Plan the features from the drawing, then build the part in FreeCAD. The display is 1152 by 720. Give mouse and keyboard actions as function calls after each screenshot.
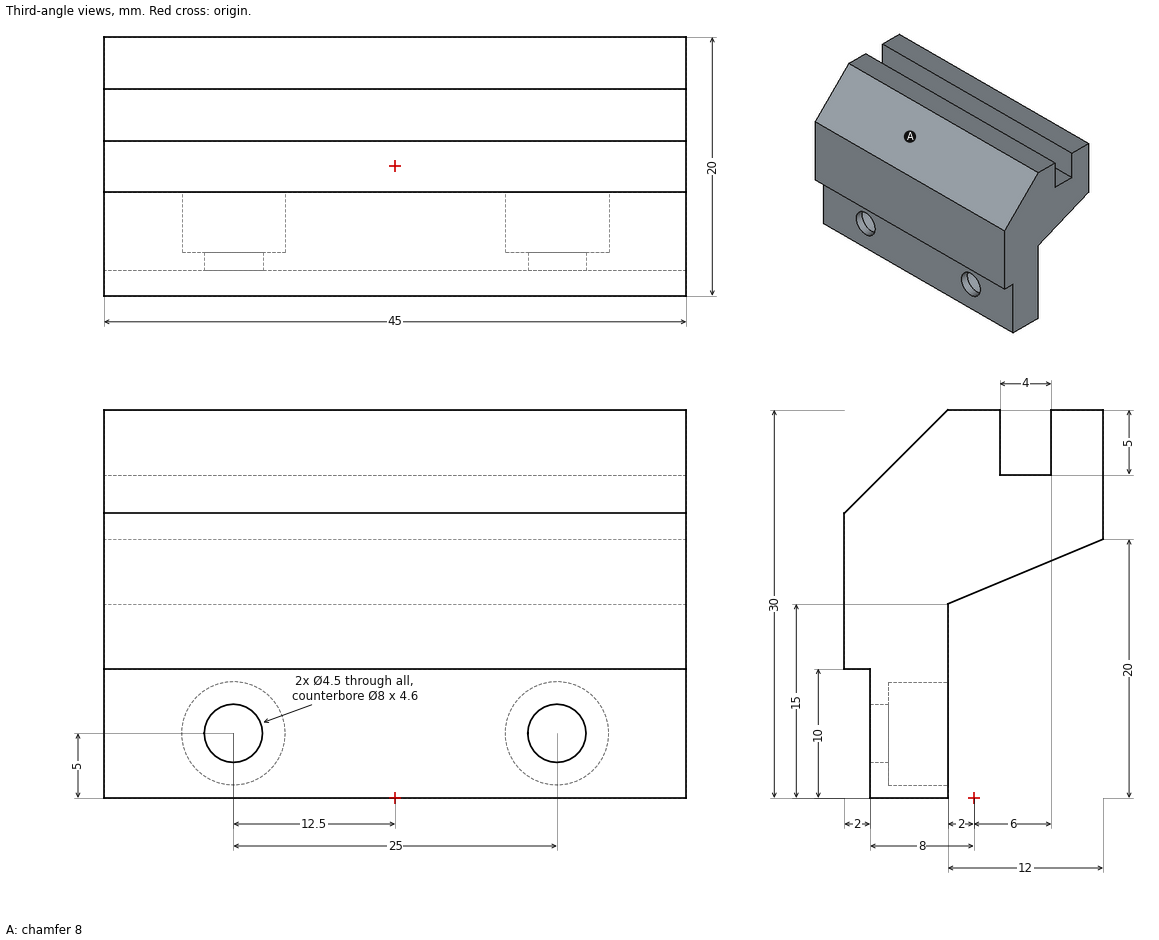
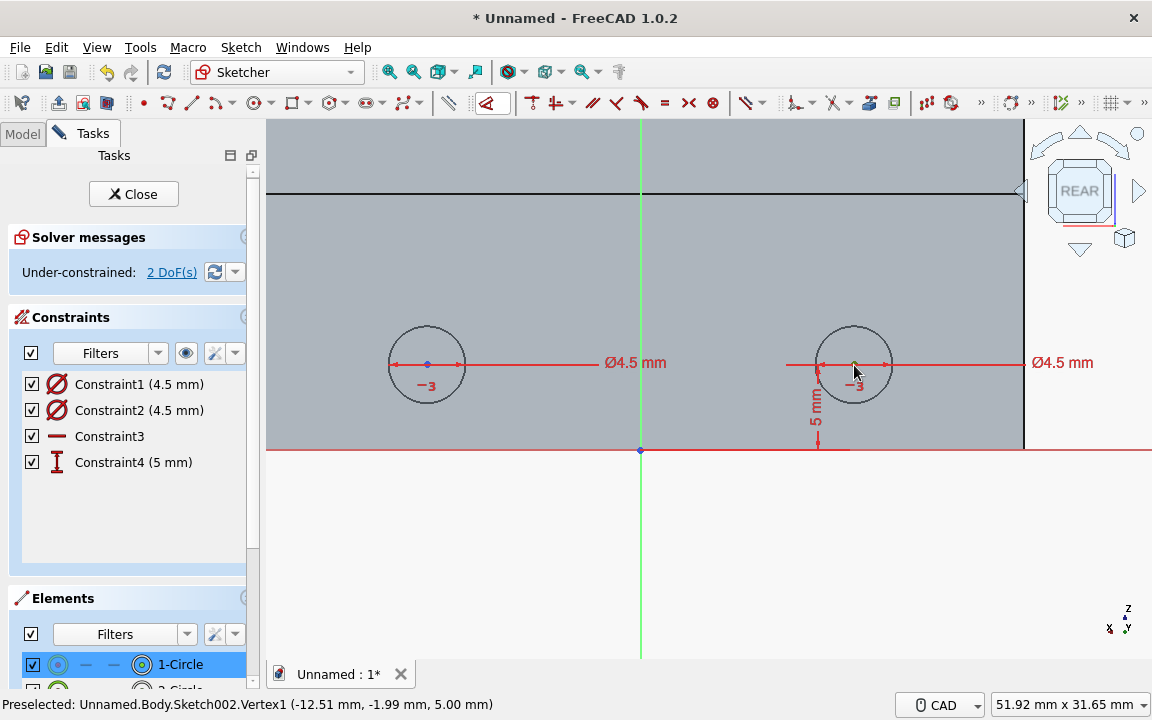
click(427, 365)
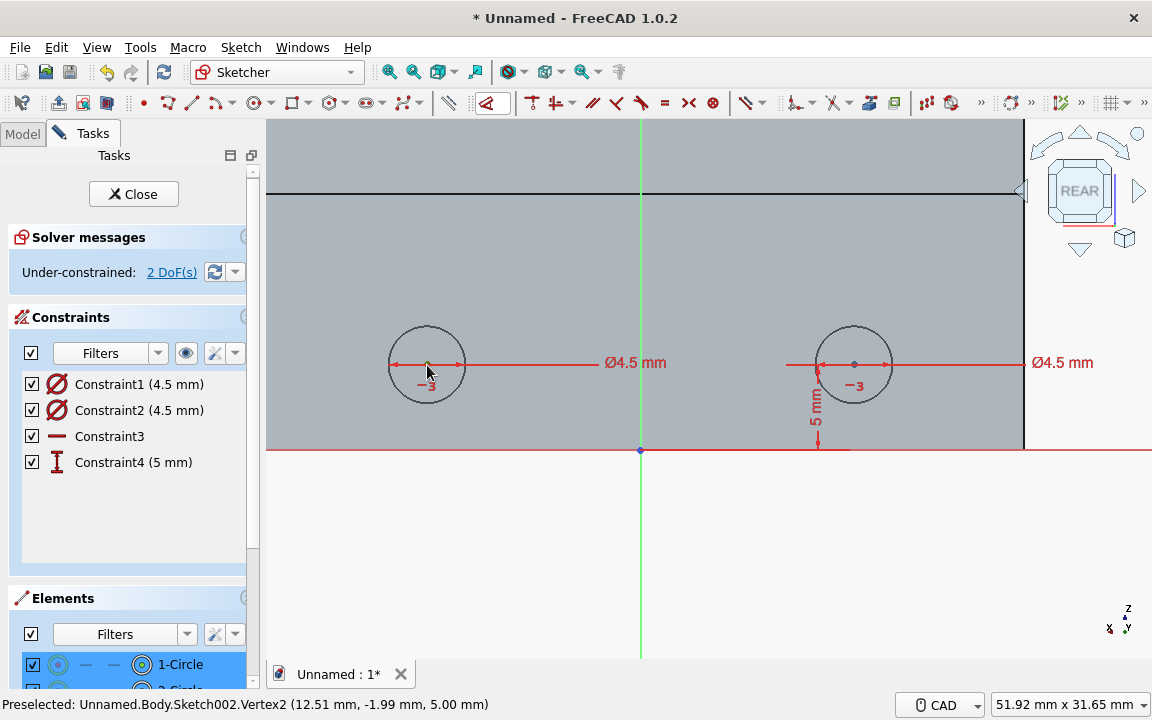
key(l)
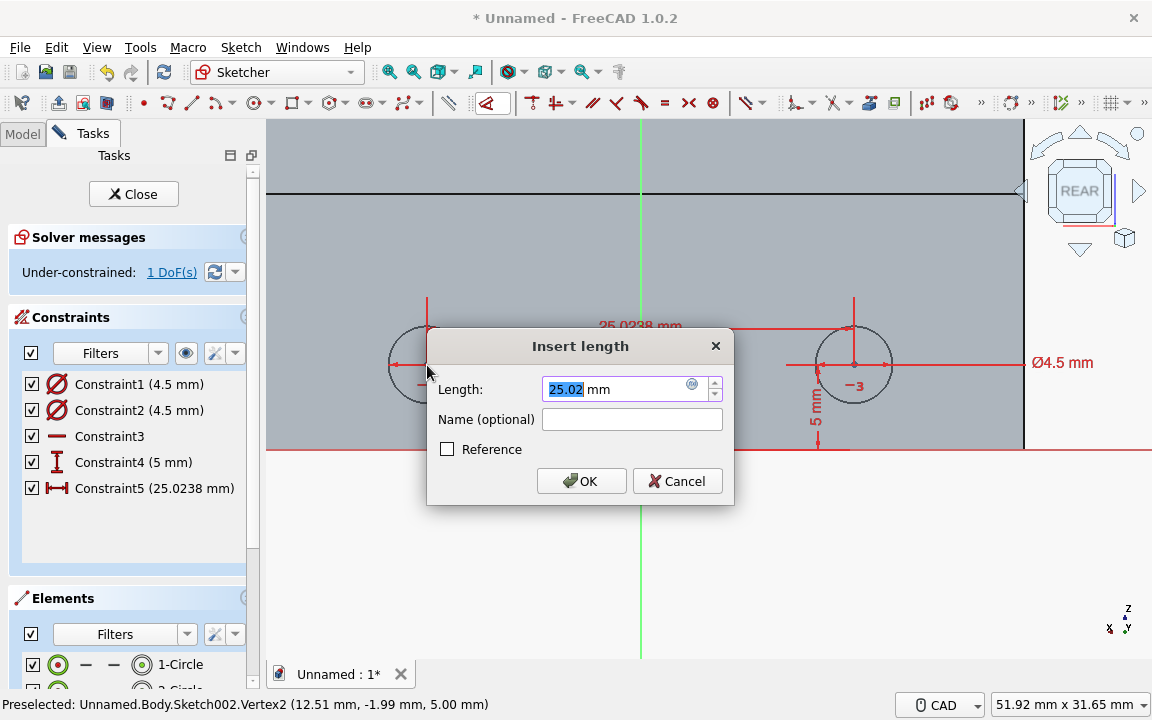
text(25)
key(Return)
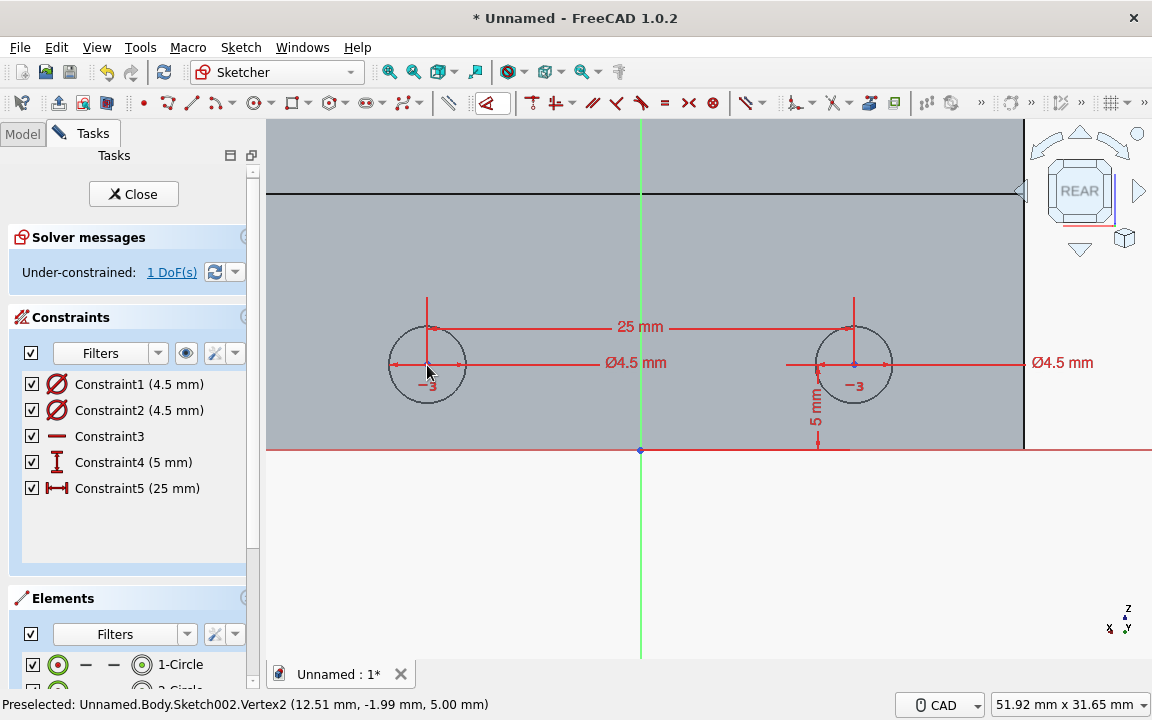
click(854, 365)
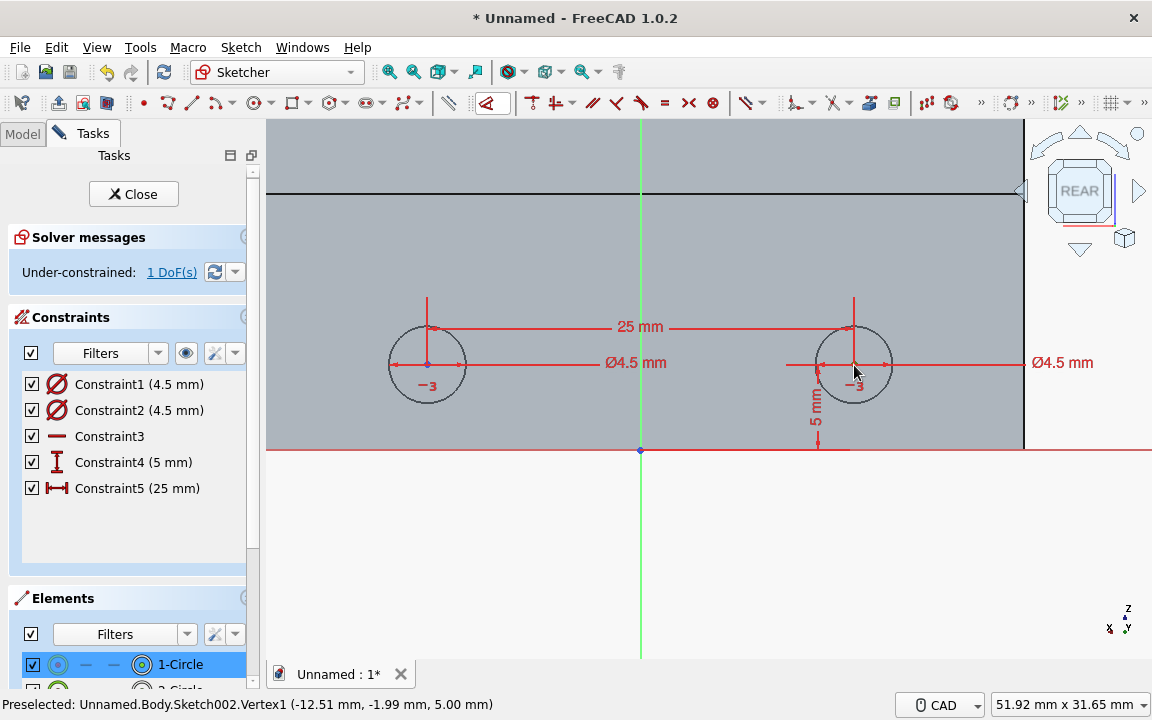
key(l)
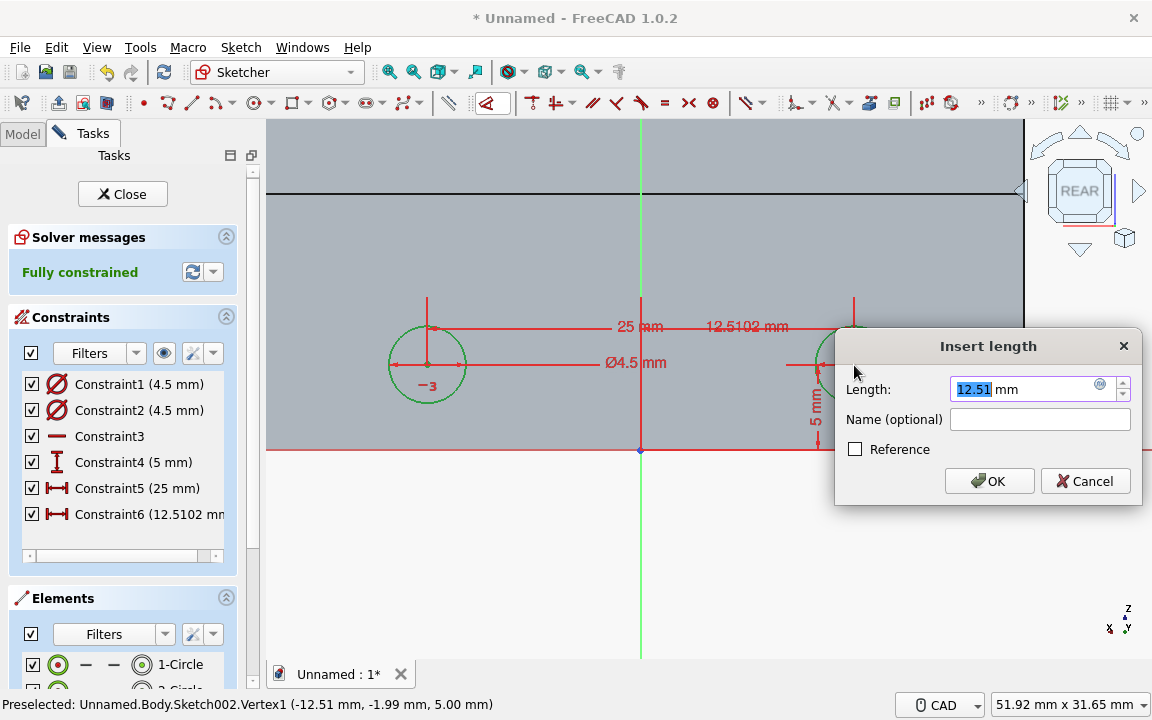
text(12.5)
key(Return)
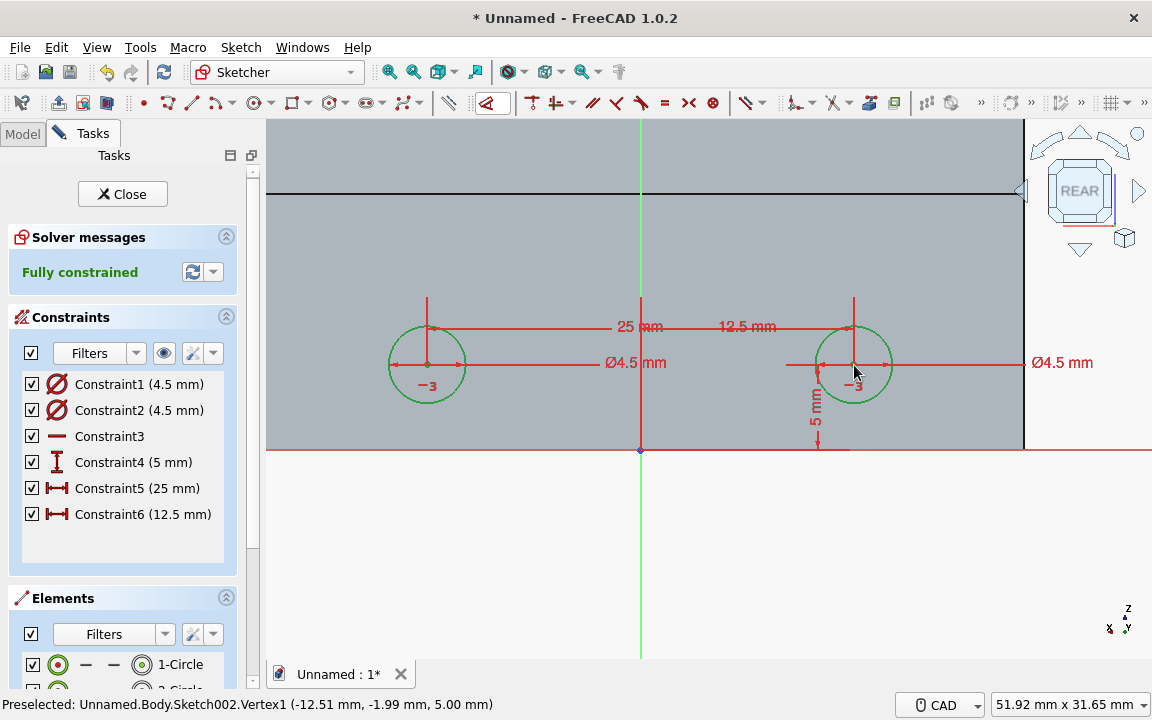
click(123, 194)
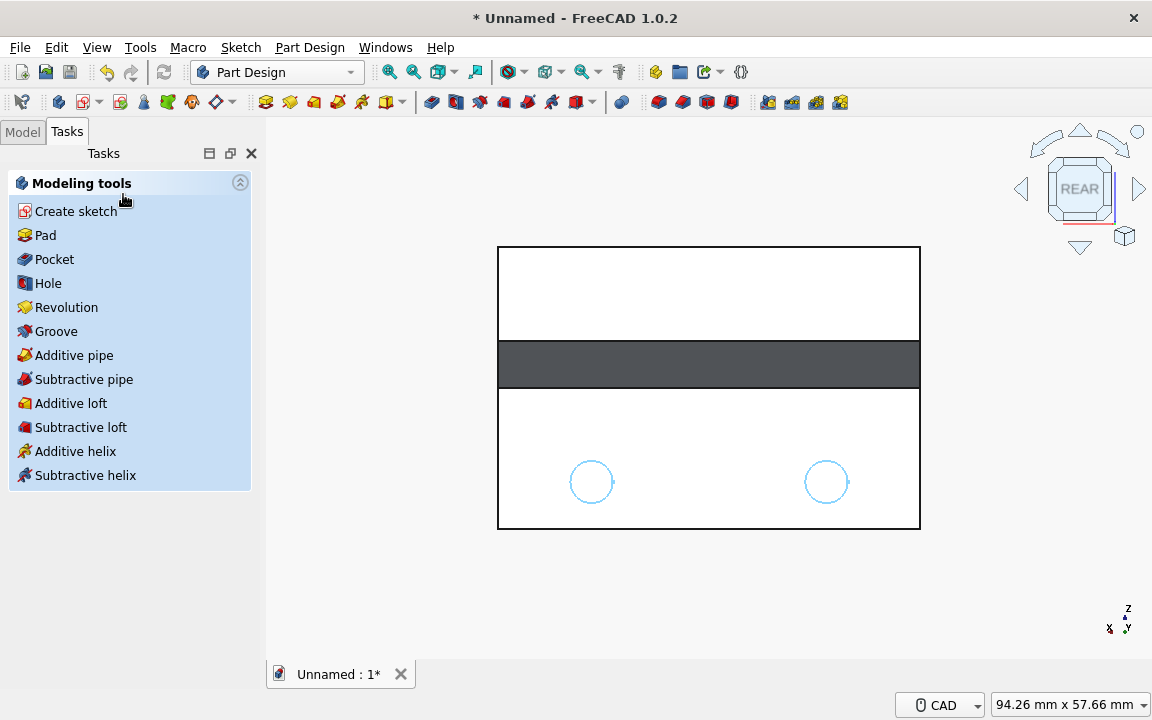
click(456, 102)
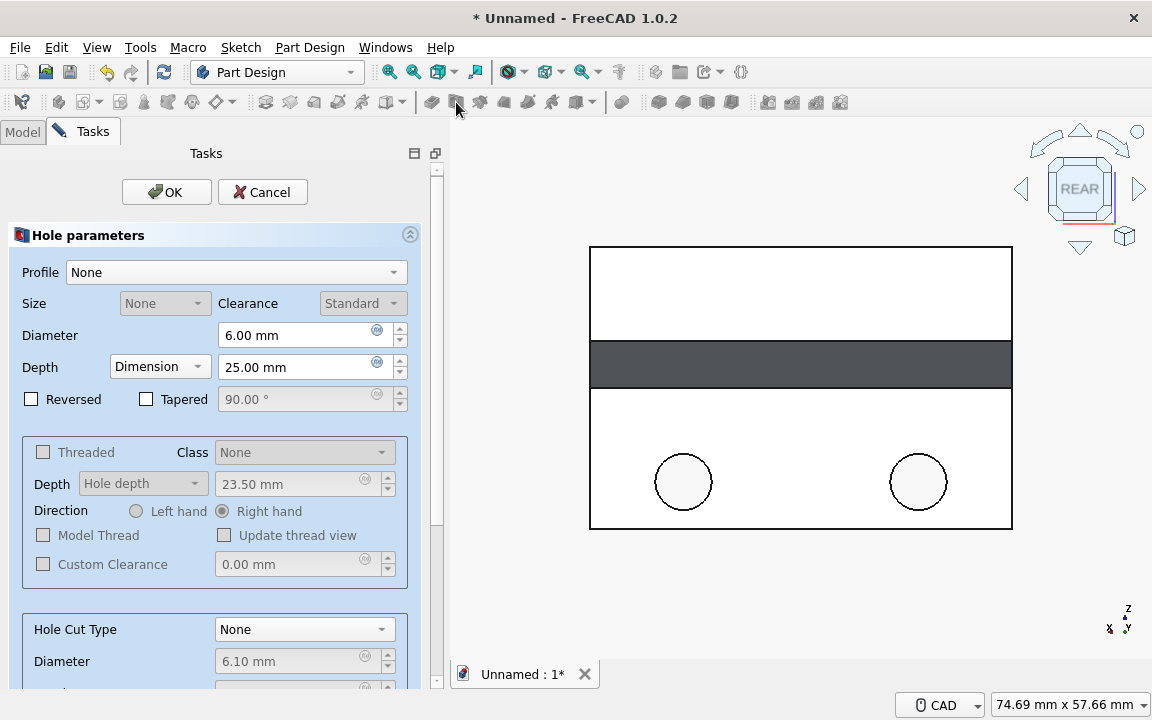
triple_click(305, 335)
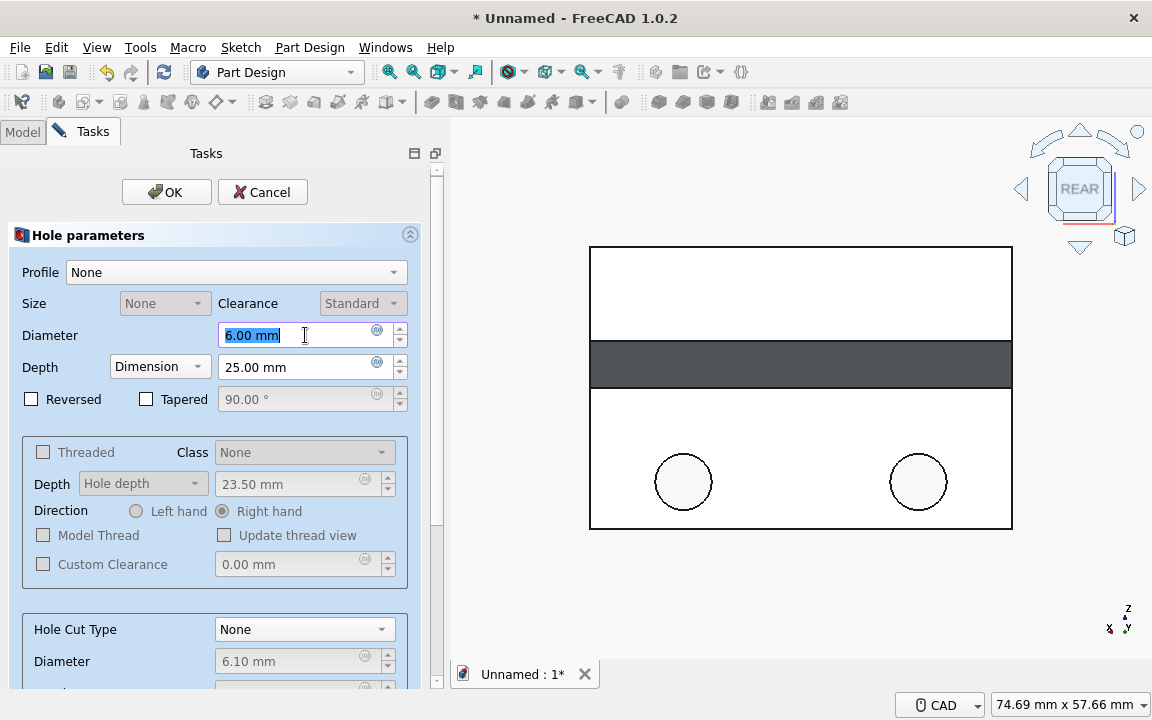
text(4.5)
key(Tab)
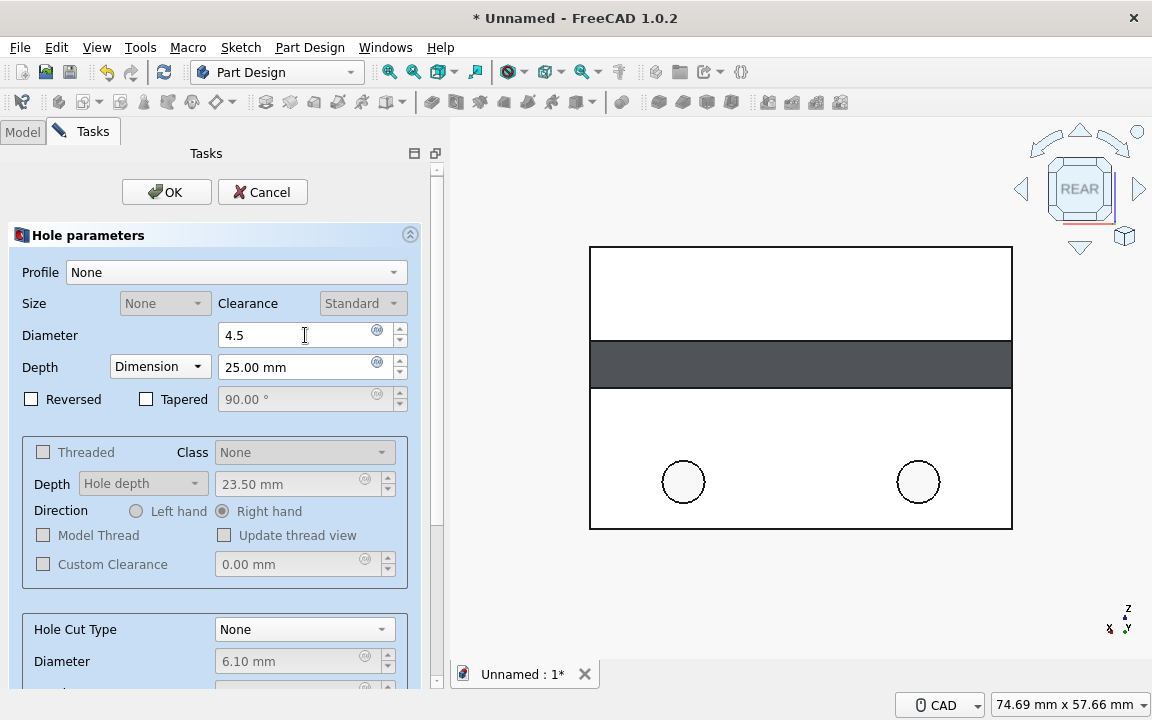
click(161, 366)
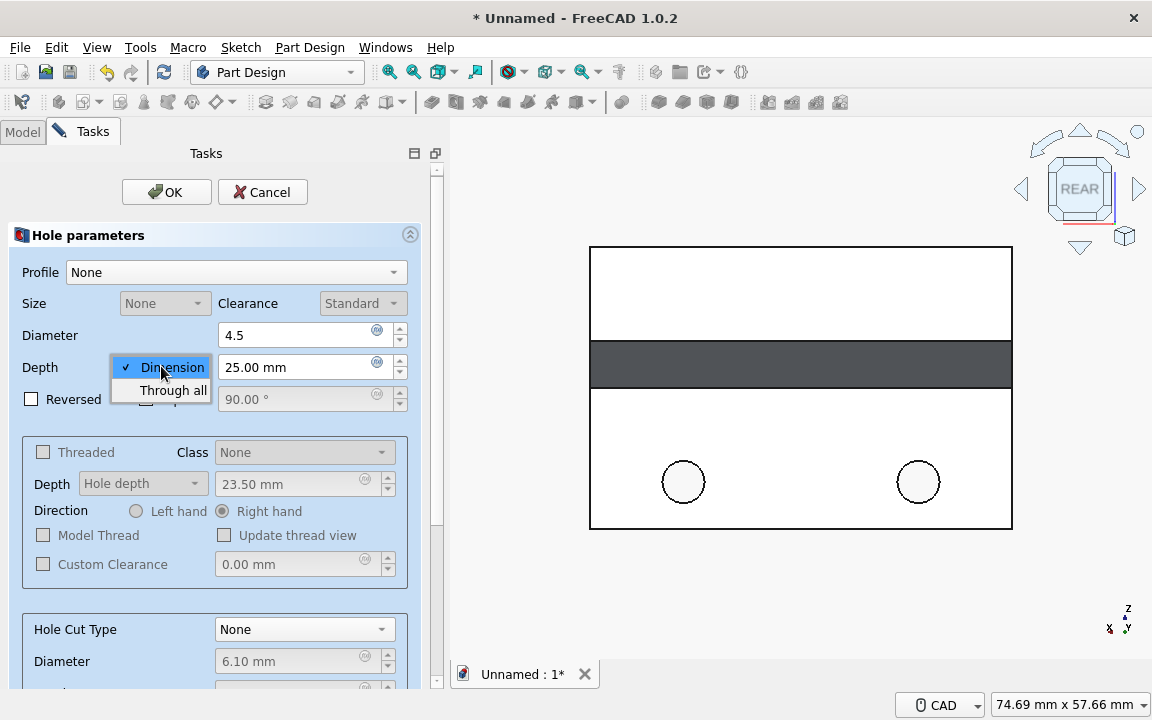
click(160, 390)